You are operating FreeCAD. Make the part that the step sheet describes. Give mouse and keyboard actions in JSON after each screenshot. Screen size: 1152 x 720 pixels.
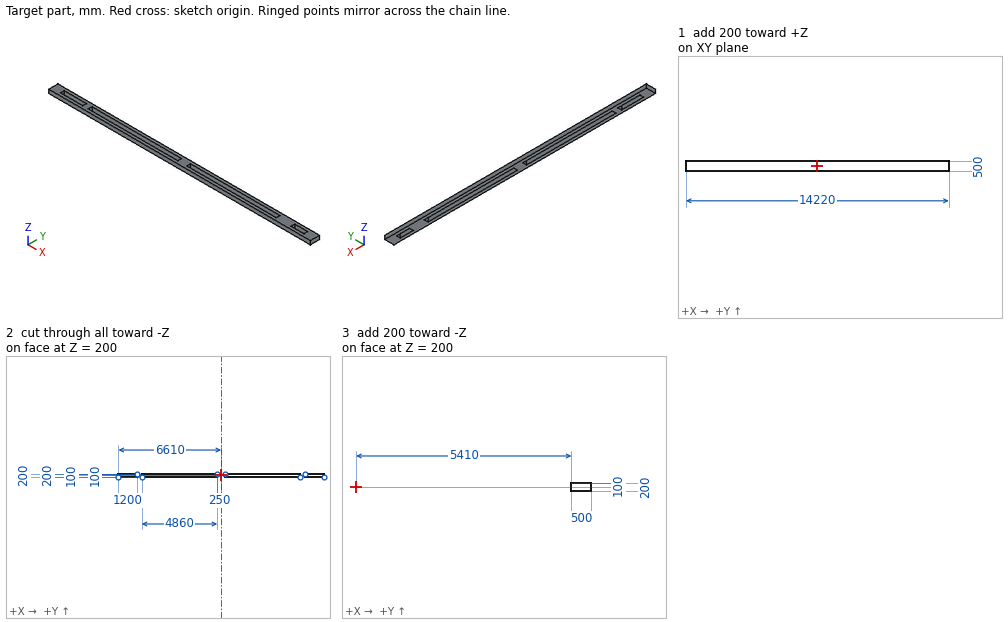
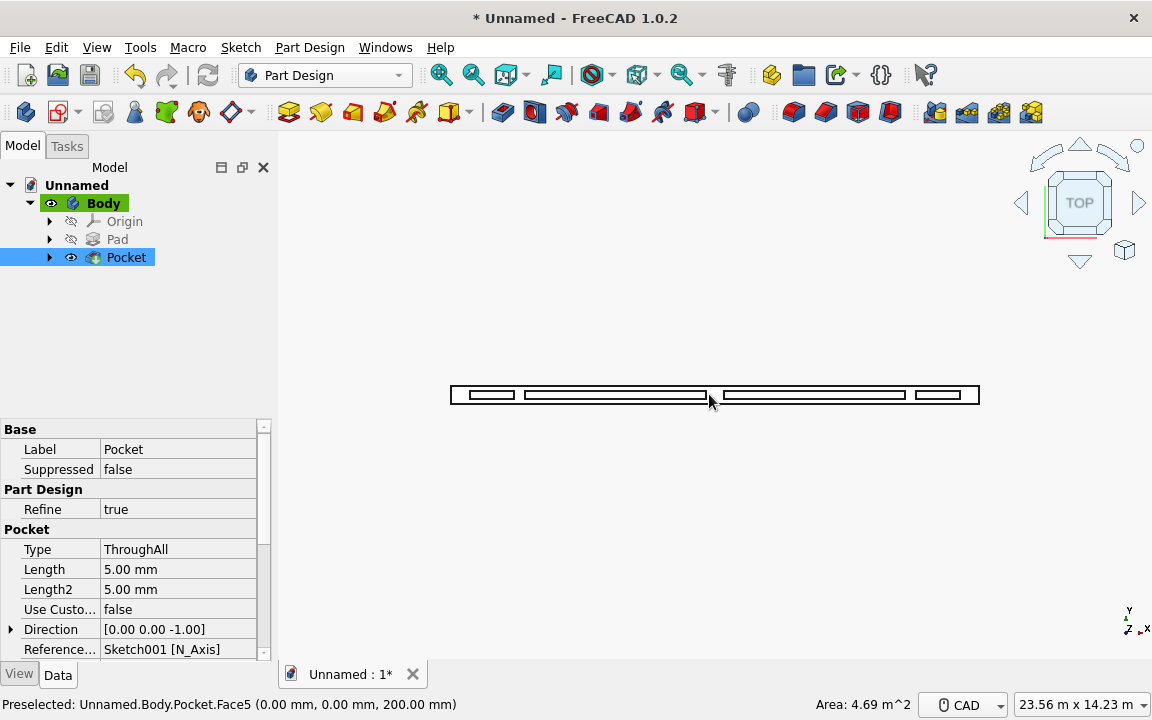
{"action": "left_click", "coordinate": [58, 112]}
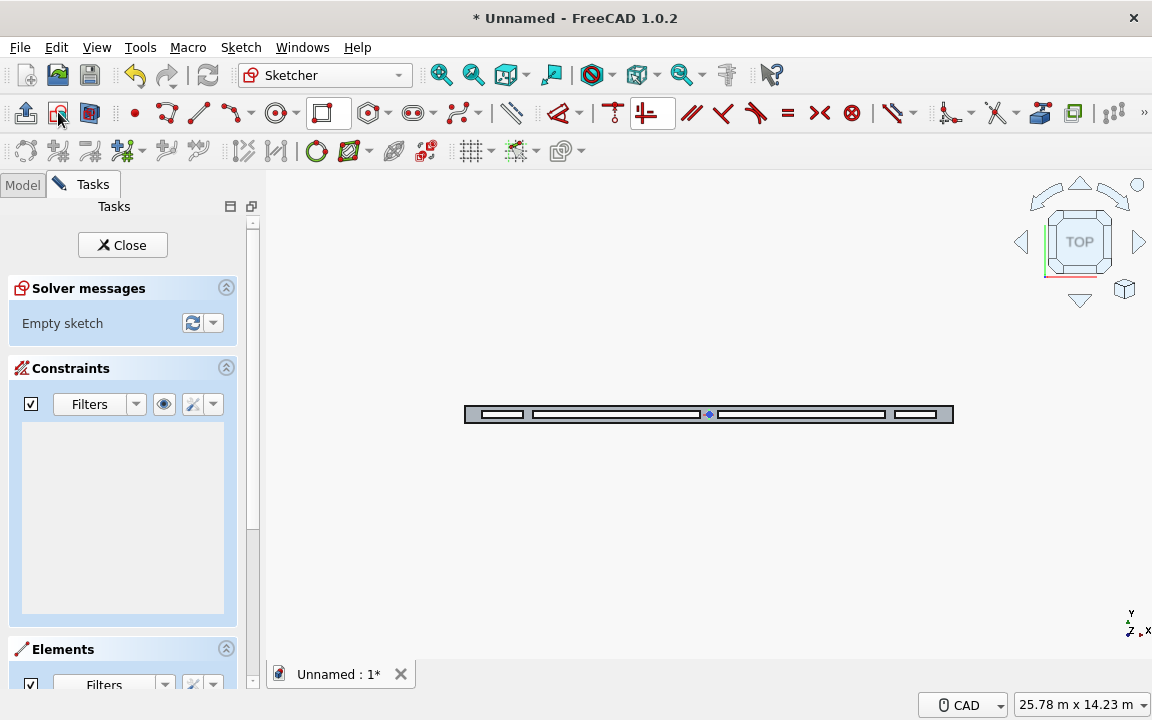
{"action": "scroll", "coordinate": [917, 414], "scroll_direction": "up", "scroll_amount": 15}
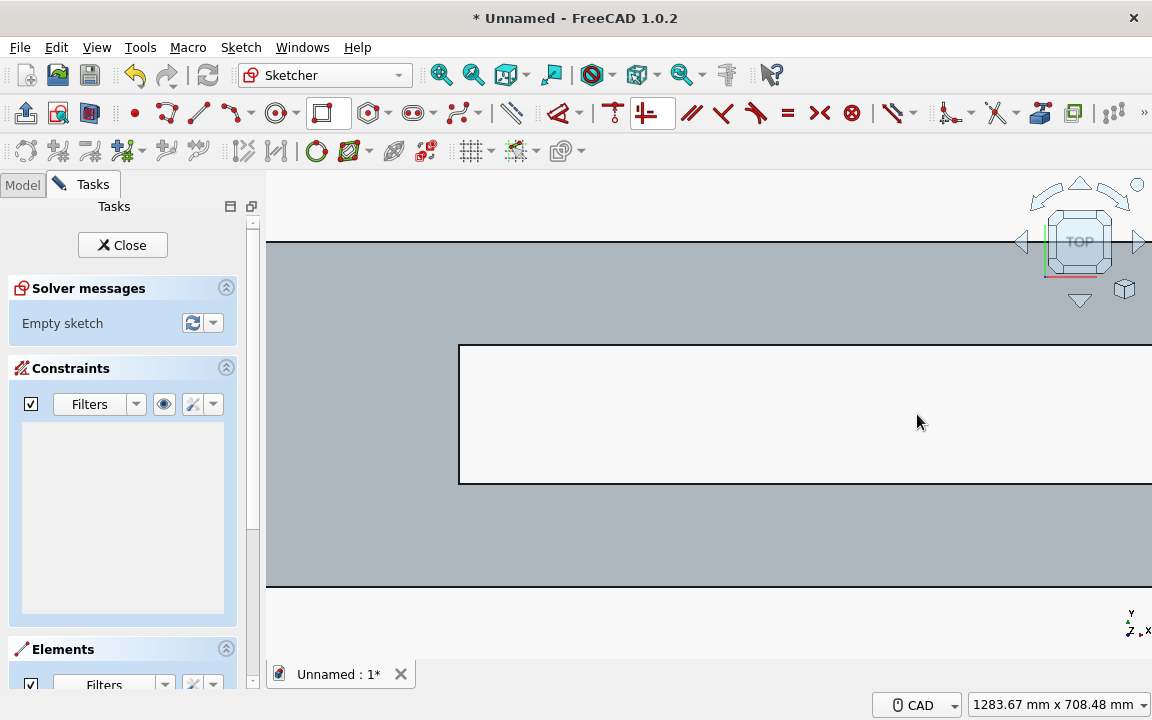
{"action": "scroll", "coordinate": [614, 414], "scroll_direction": "up", "scroll_amount": 2}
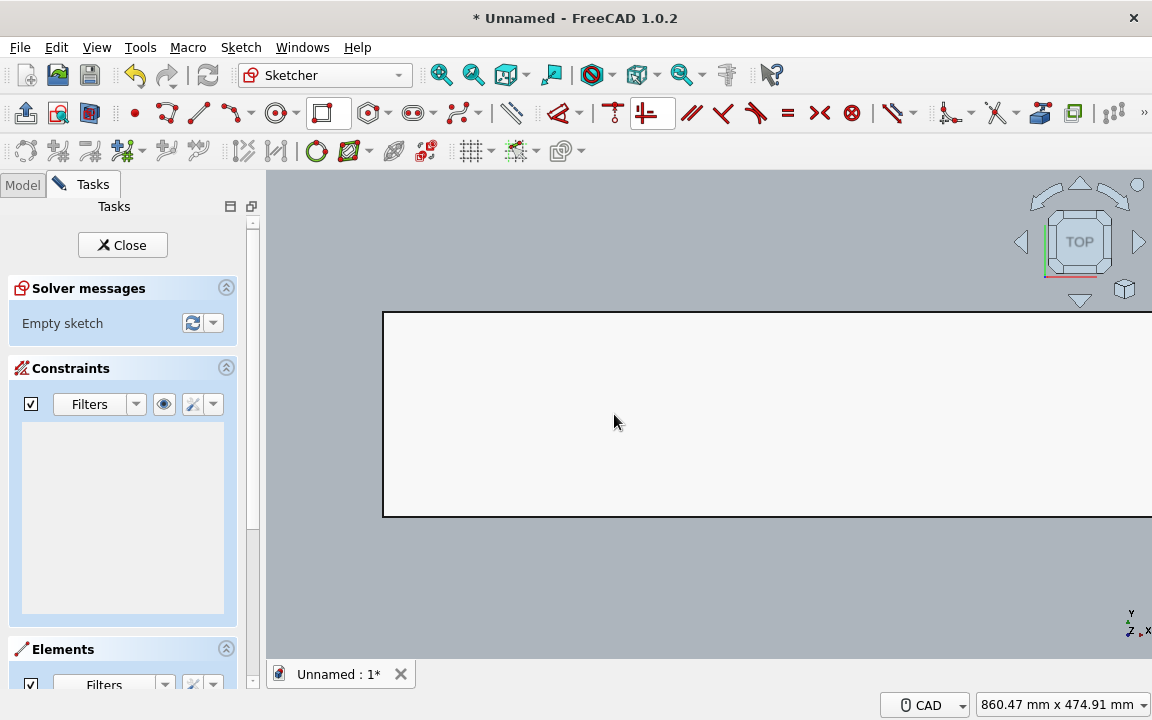
{"action": "left_click", "coordinate": [322, 114]}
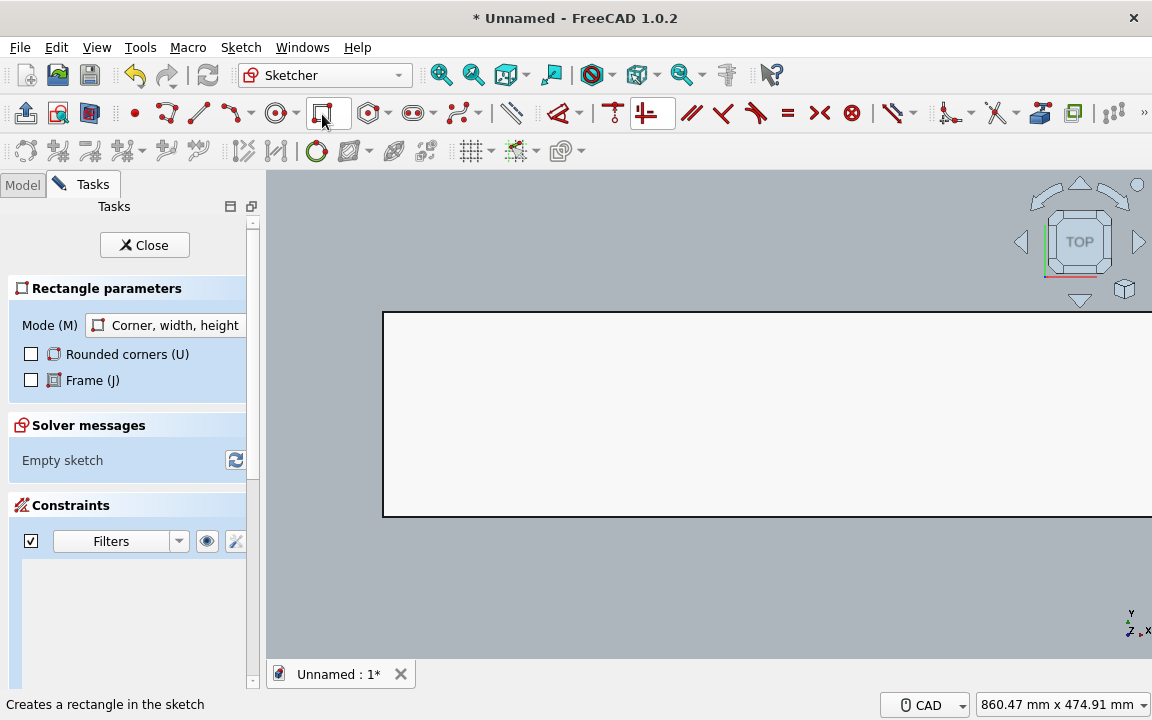
{"action": "left_click", "coordinate": [383, 312]}
{"action": "mouse_move", "coordinate": [898, 517]}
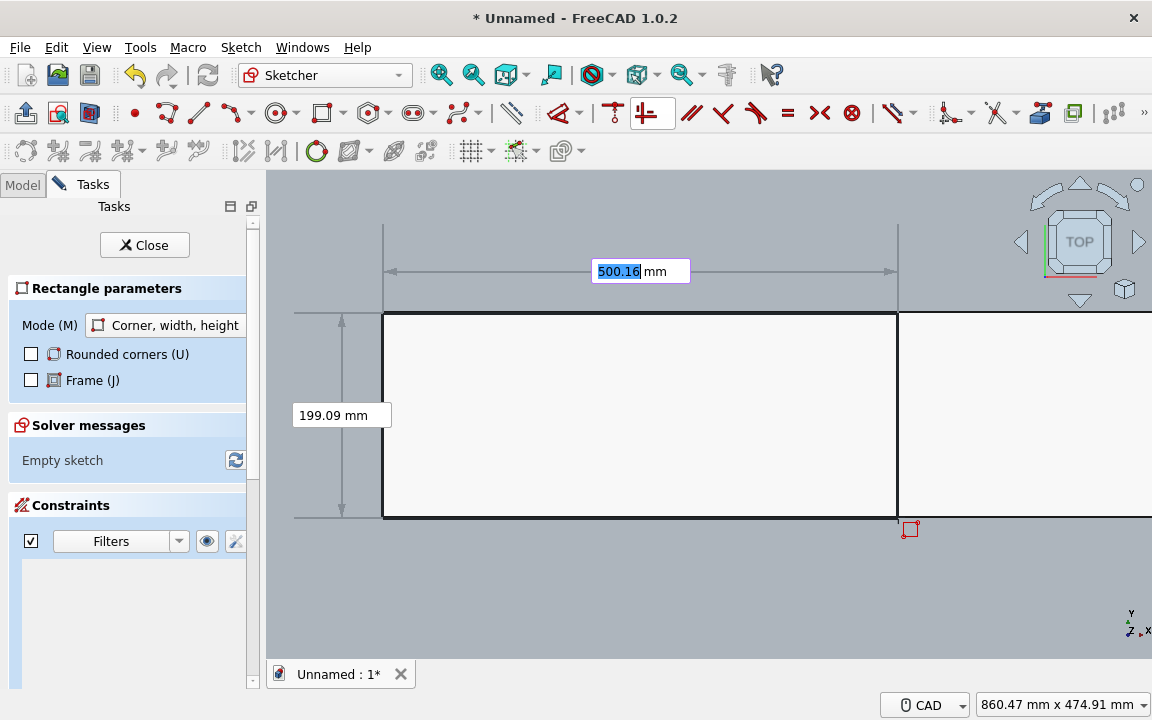
{"action": "type", "text": "500"}
{"action": "key", "text": "Tab"}
{"action": "type", "text": "200"}
{"action": "key", "text": "Return"}
{"action": "key", "text": "Escape"}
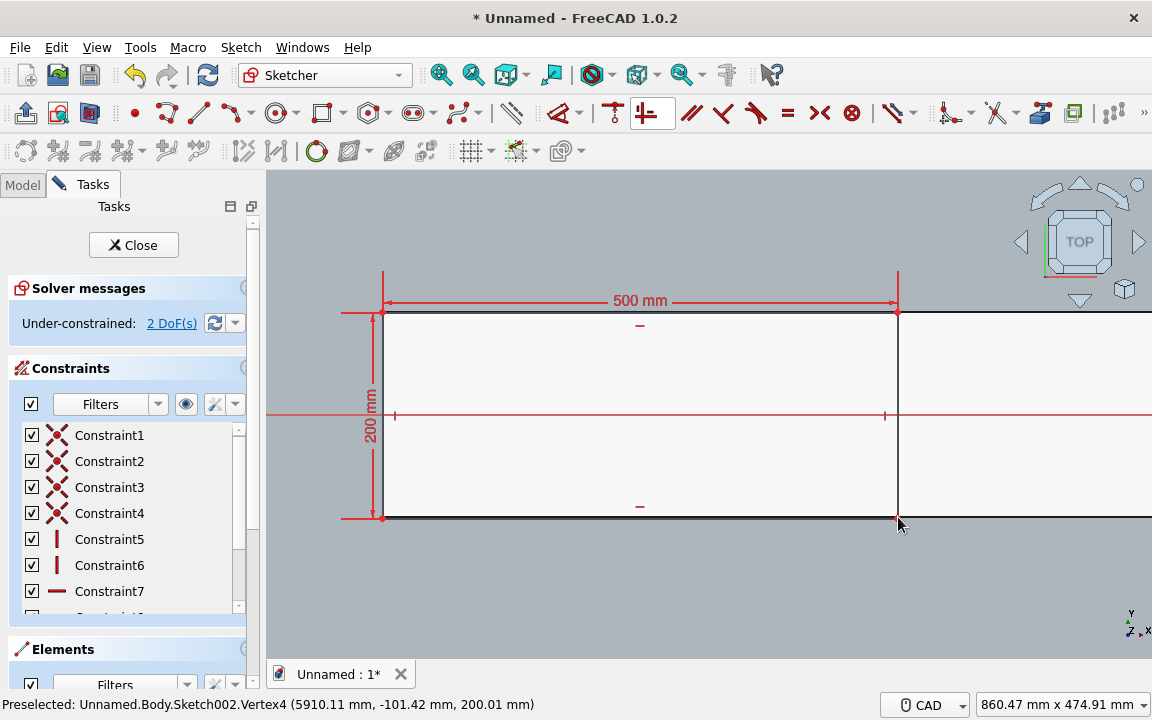
{"action": "left_click", "coordinate": [558, 114]}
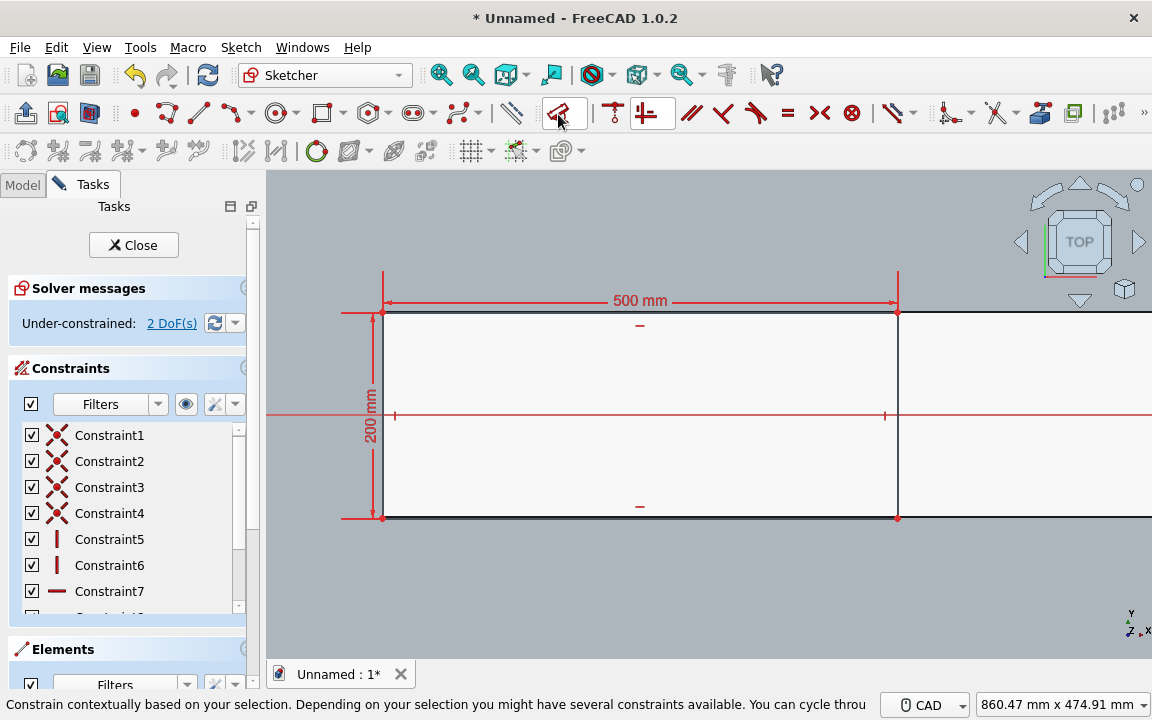
{"action": "left_click", "coordinate": [383, 313]}
{"action": "left_click", "coordinate": [417, 364]}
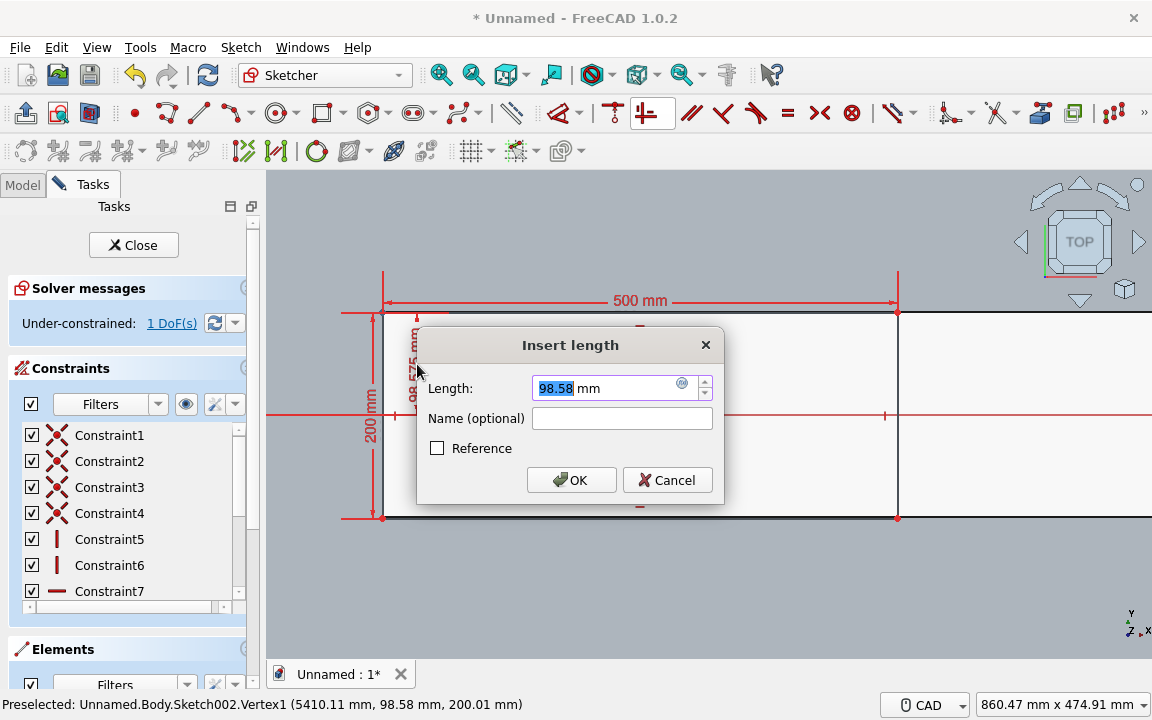
{"action": "type", "text": "100"}
{"action": "key", "text": "Return"}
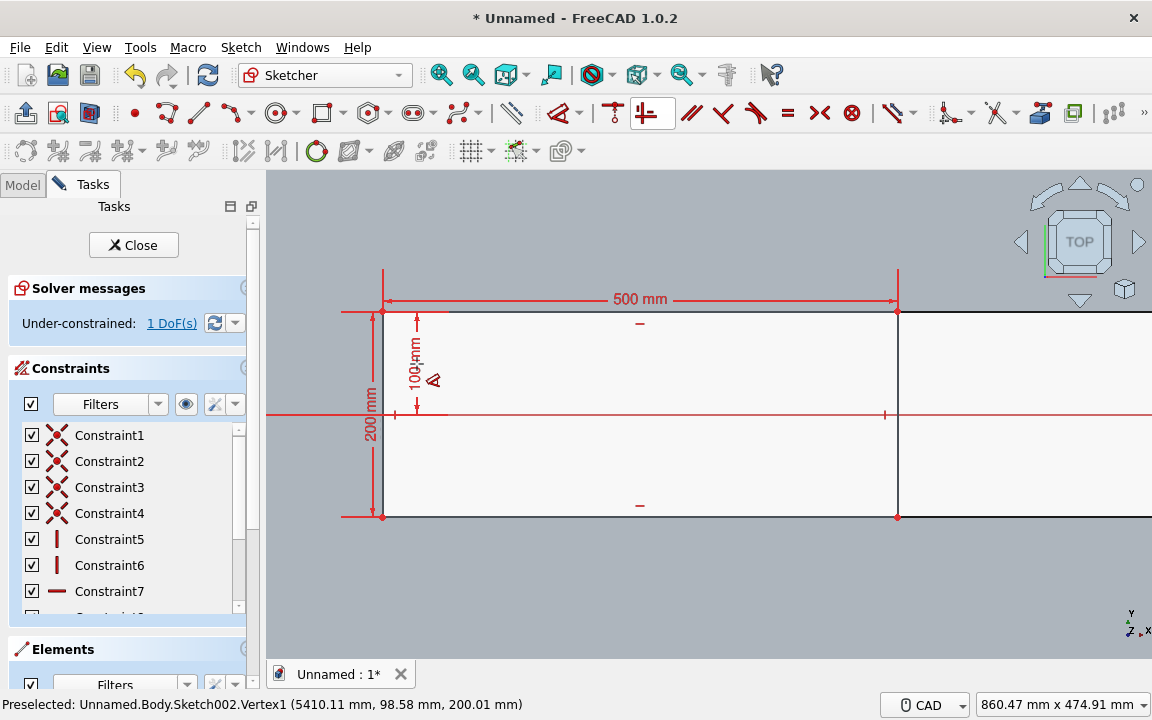
{"action": "left_click", "coordinate": [383, 312]}
{"action": "left_click", "coordinate": [339, 278]}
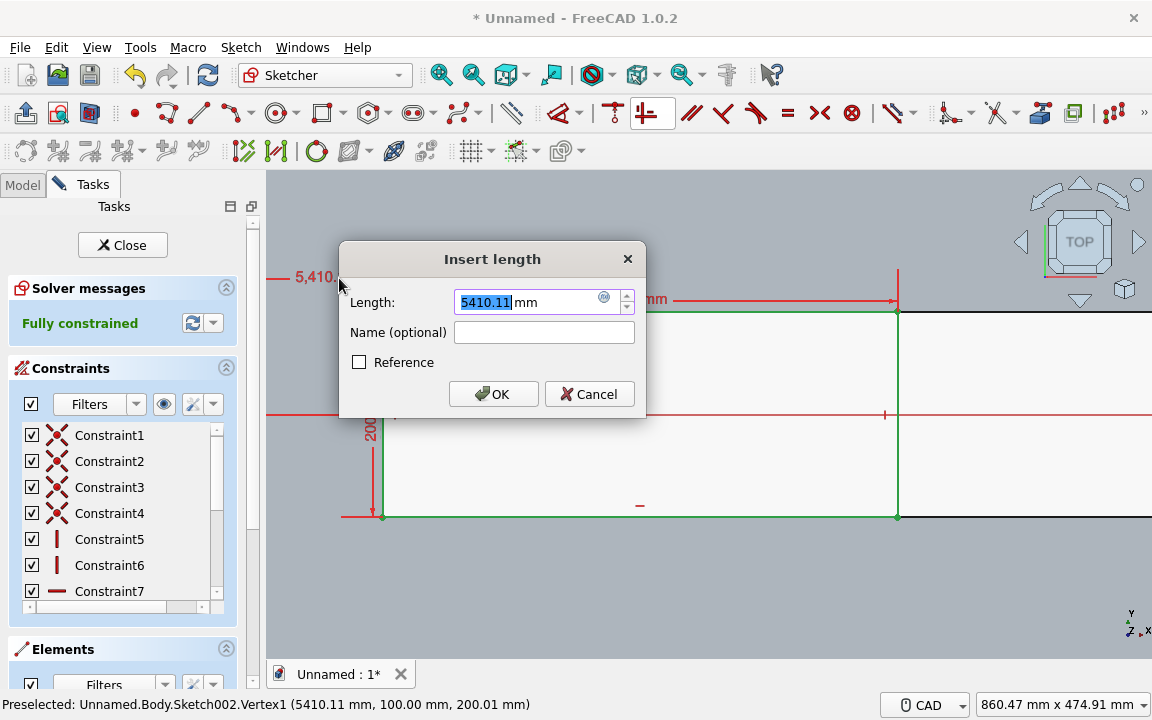
{"action": "type", "text": "5410"}
{"action": "key", "text": "Return"}
{"action": "key", "text": "Escape"}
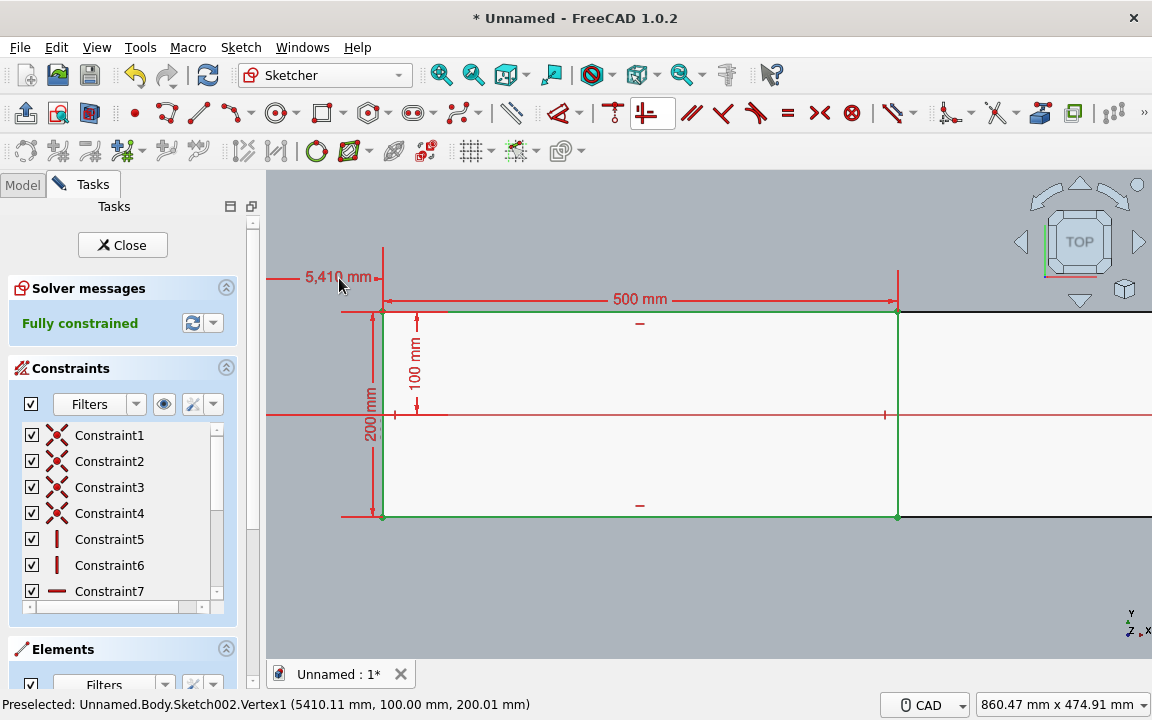
{"action": "left_click", "coordinate": [123, 245]}